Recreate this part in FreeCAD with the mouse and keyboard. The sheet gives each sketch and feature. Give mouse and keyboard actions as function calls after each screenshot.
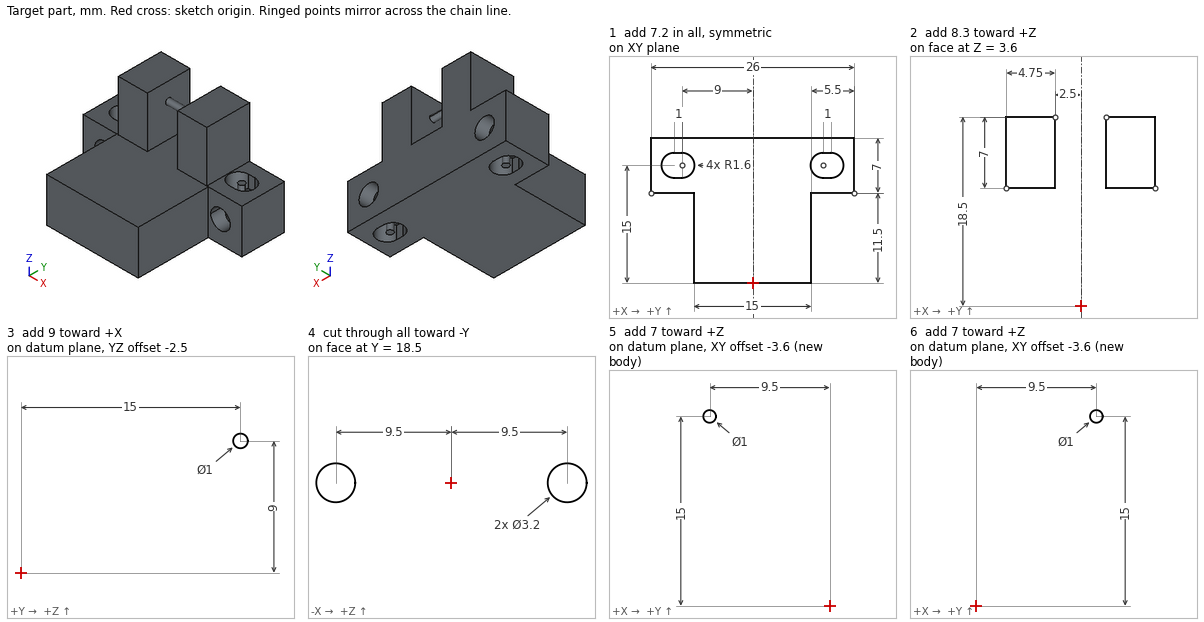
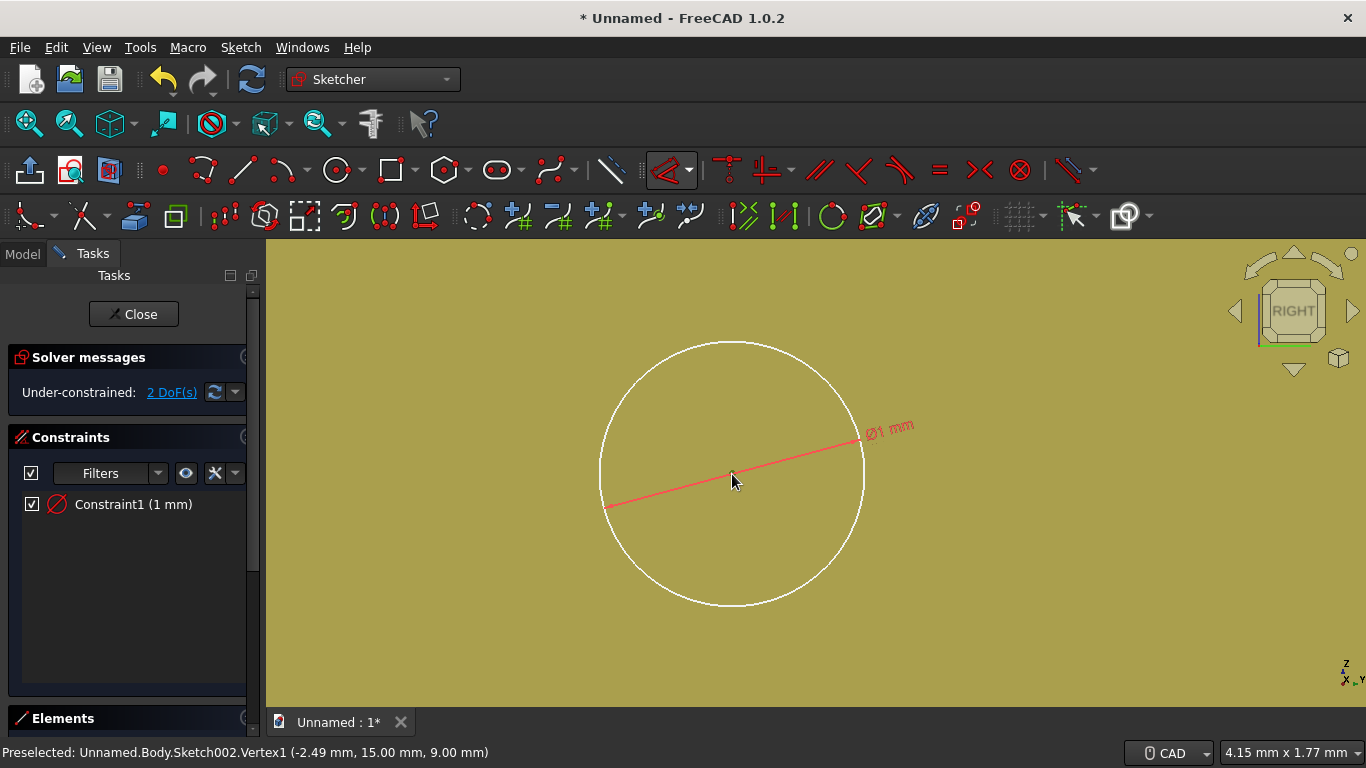
key(i)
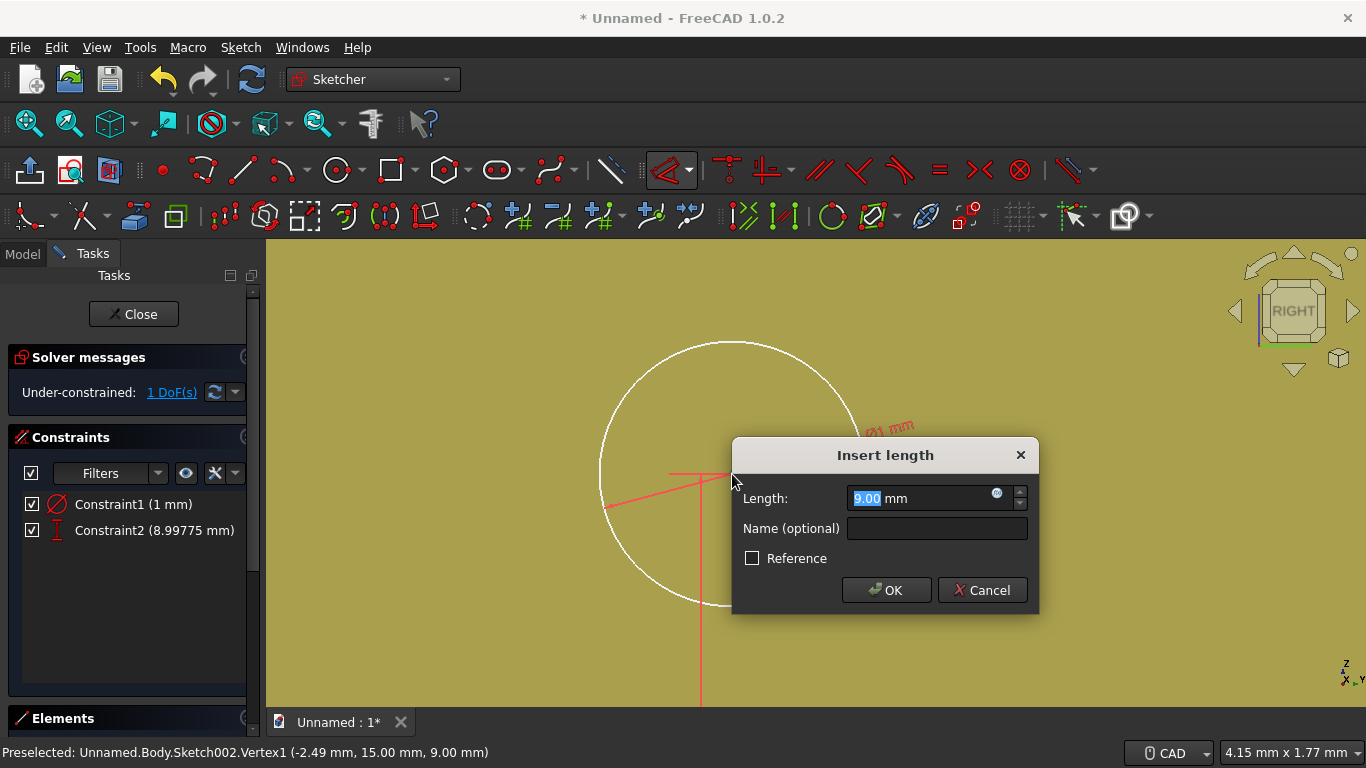
text(9)
key(Return)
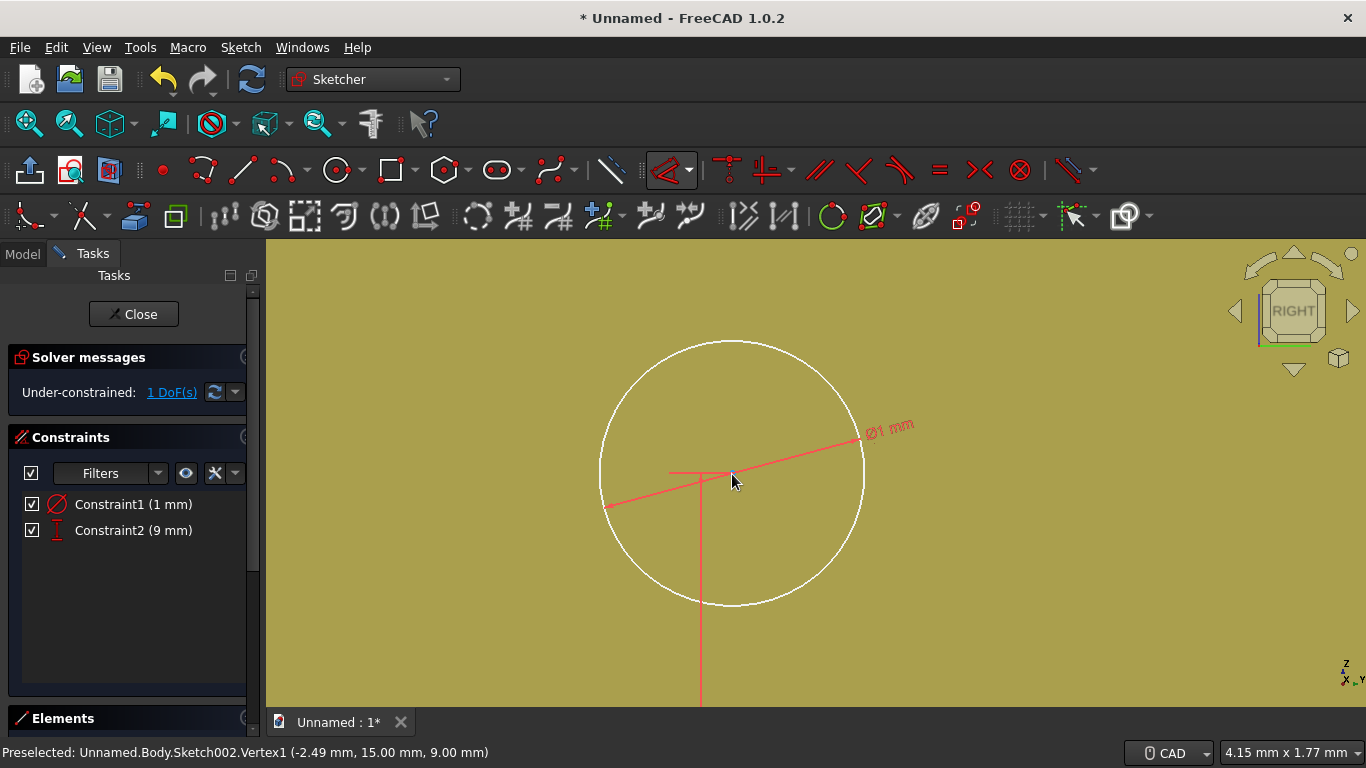
click(732, 473)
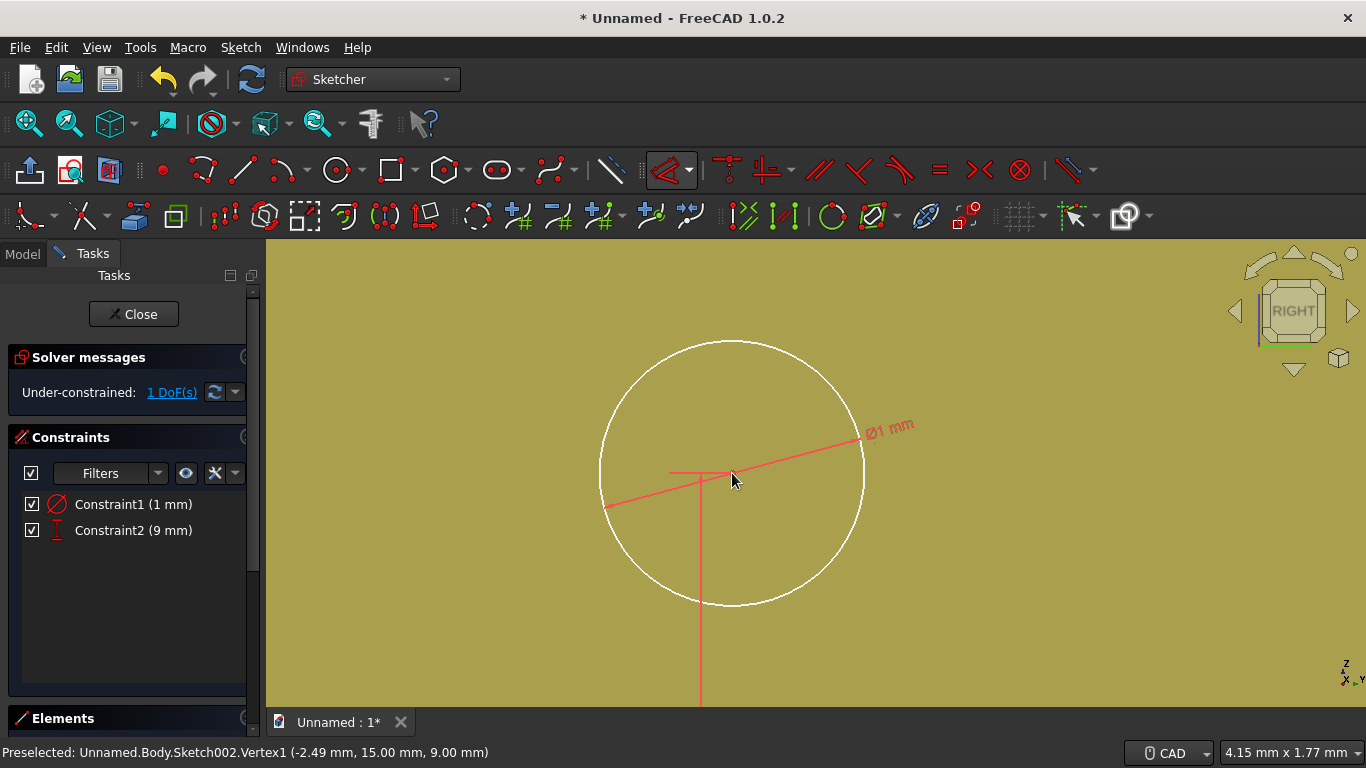
key(l)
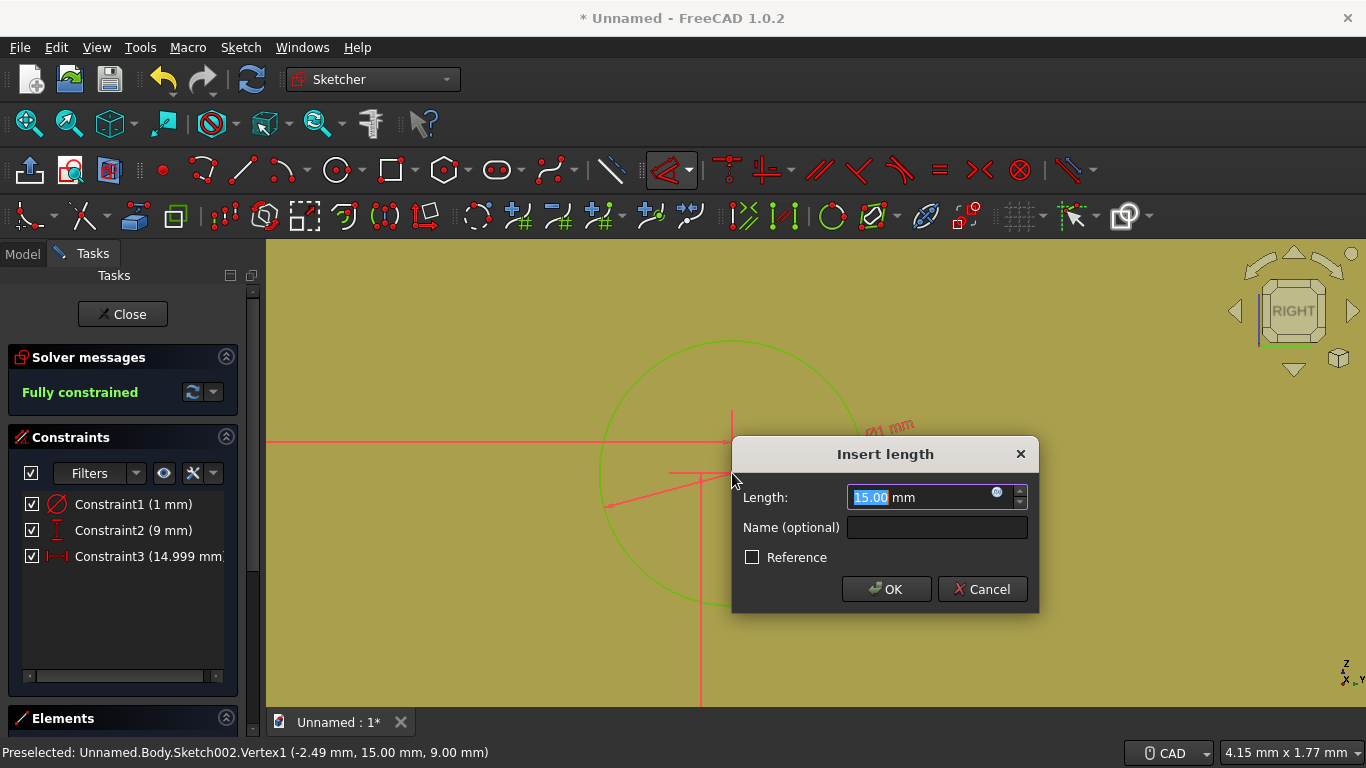
text(15)
key(Return)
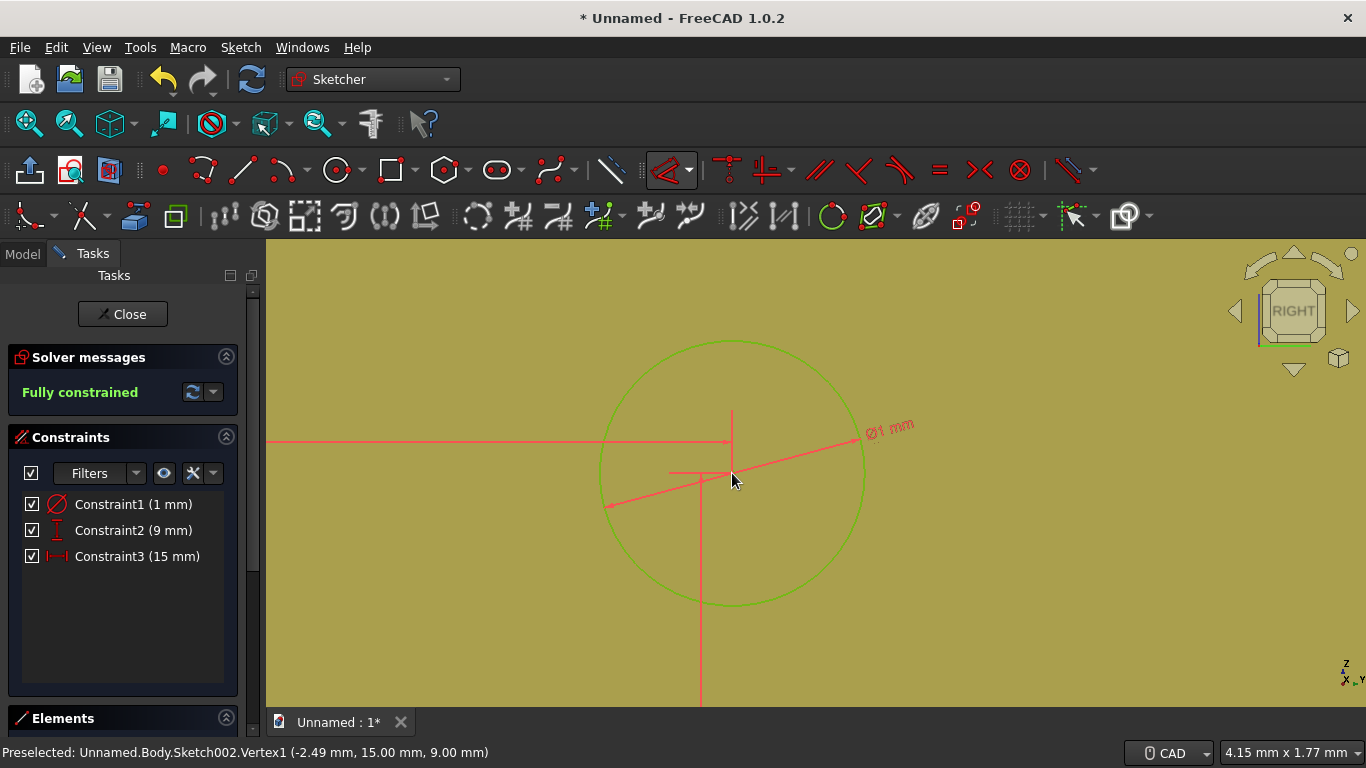
click(123, 314)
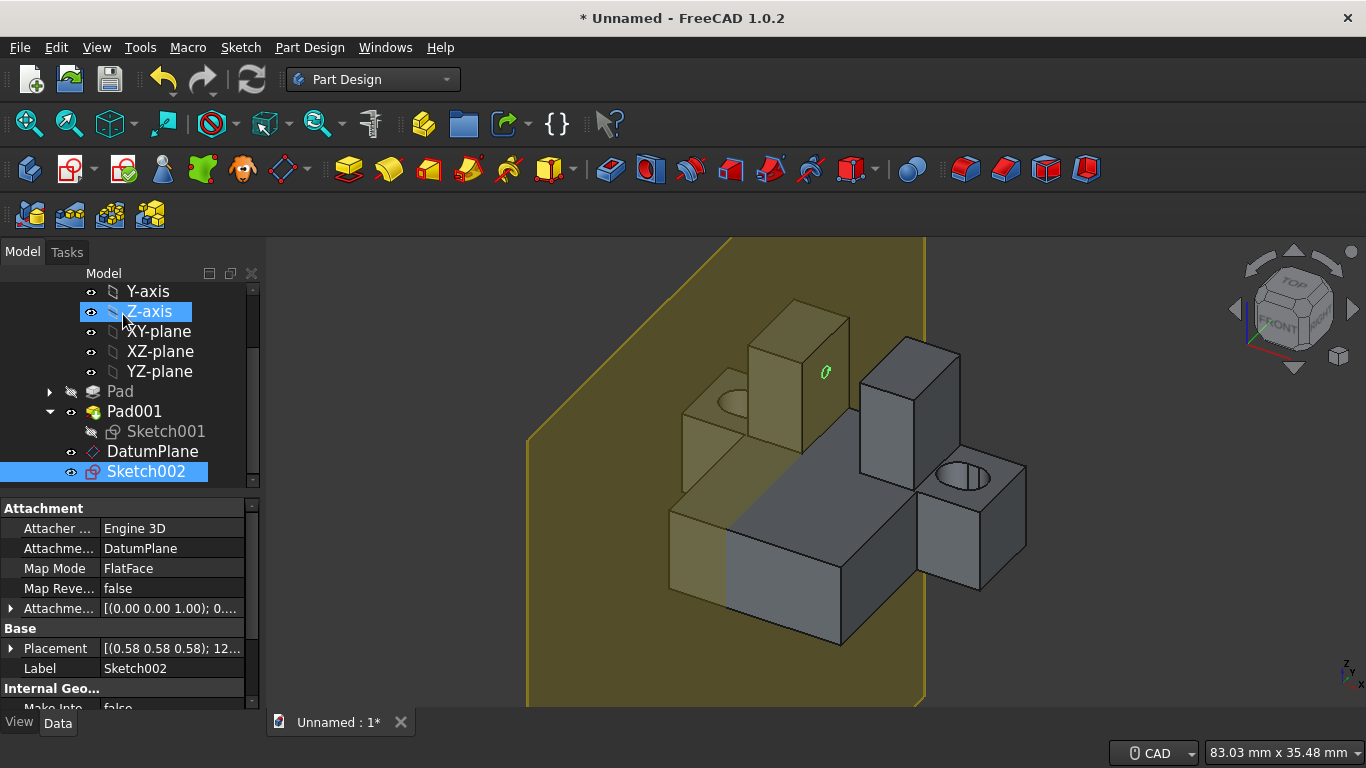
click(350, 170)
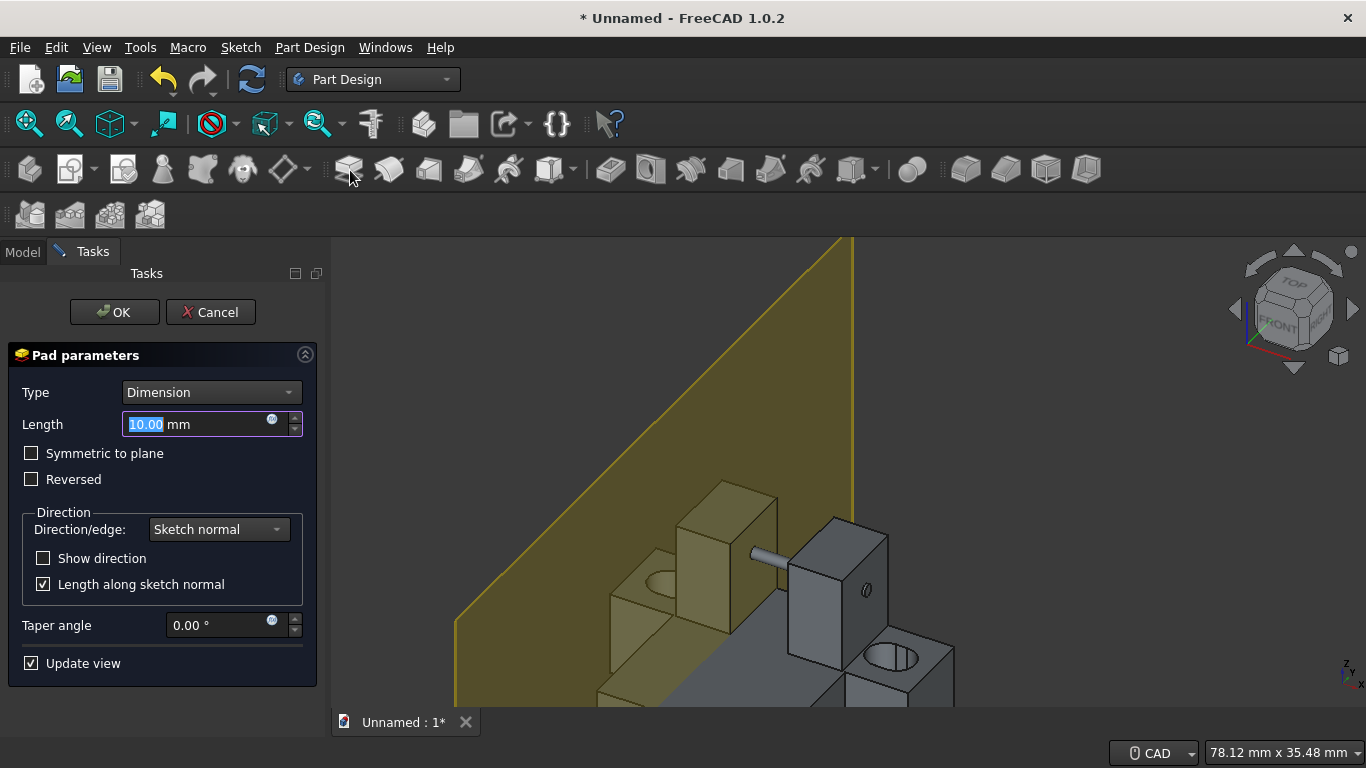
text(9)
key(Tab)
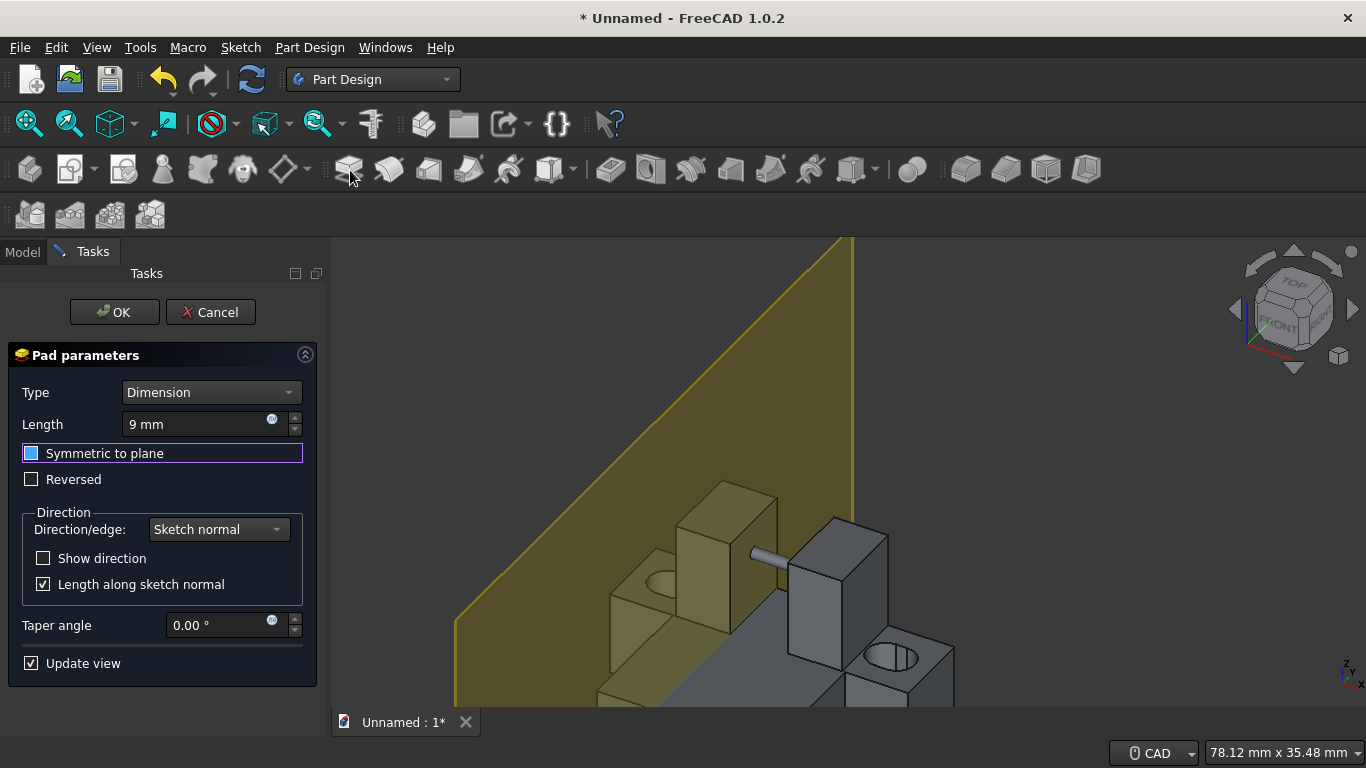
click(115, 312)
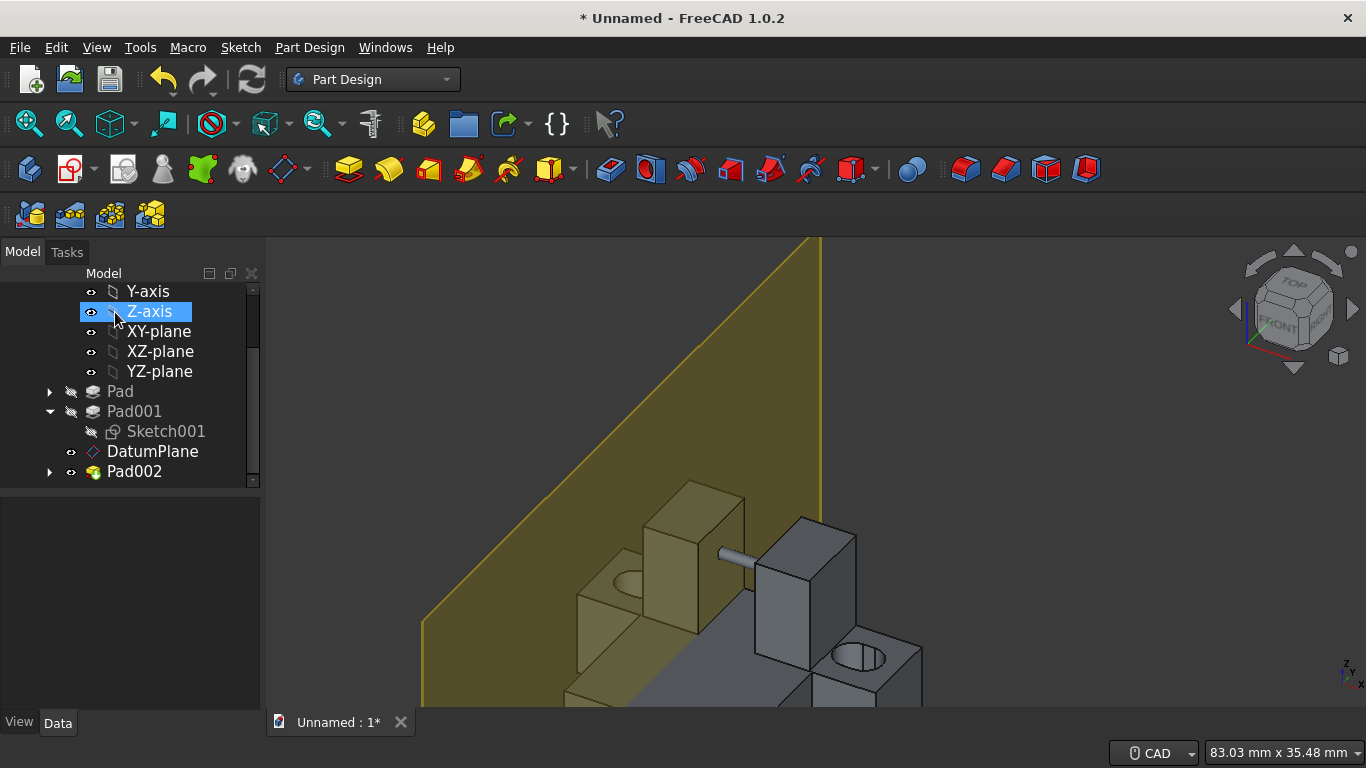
click(116, 452)
key(space)